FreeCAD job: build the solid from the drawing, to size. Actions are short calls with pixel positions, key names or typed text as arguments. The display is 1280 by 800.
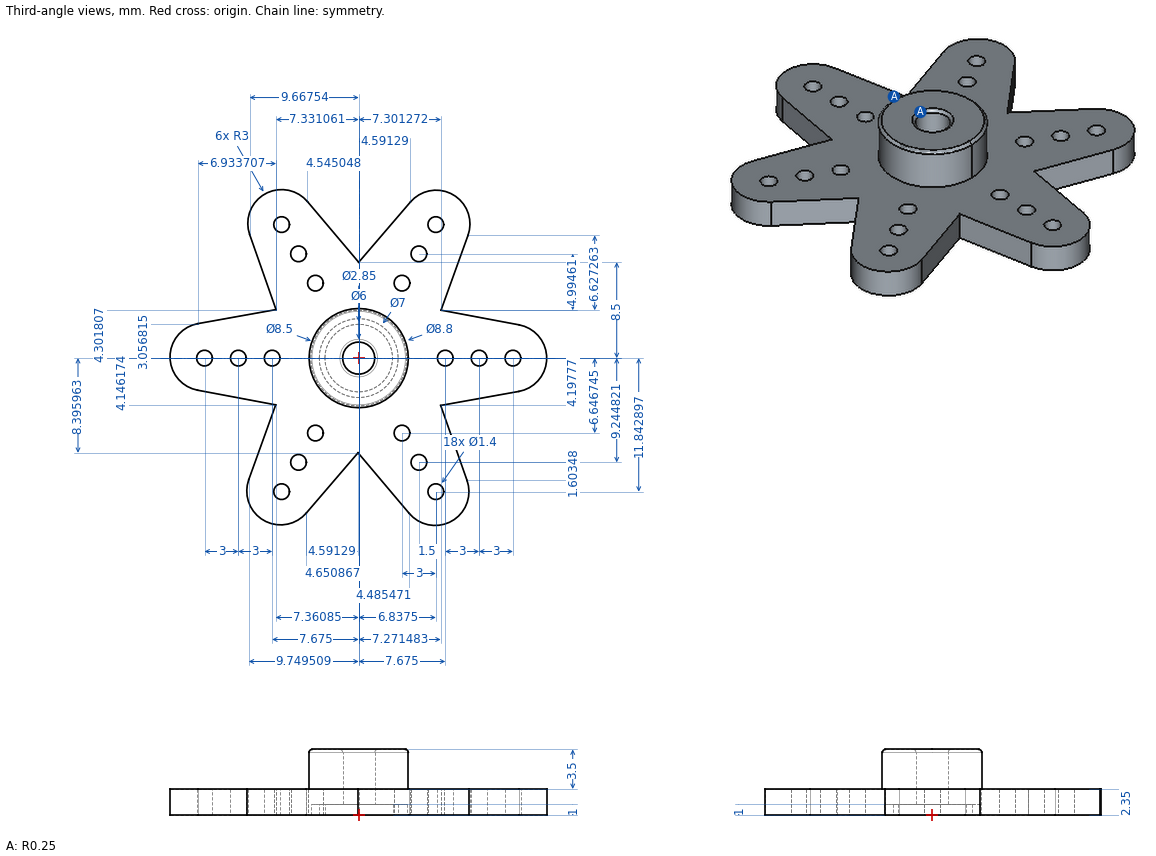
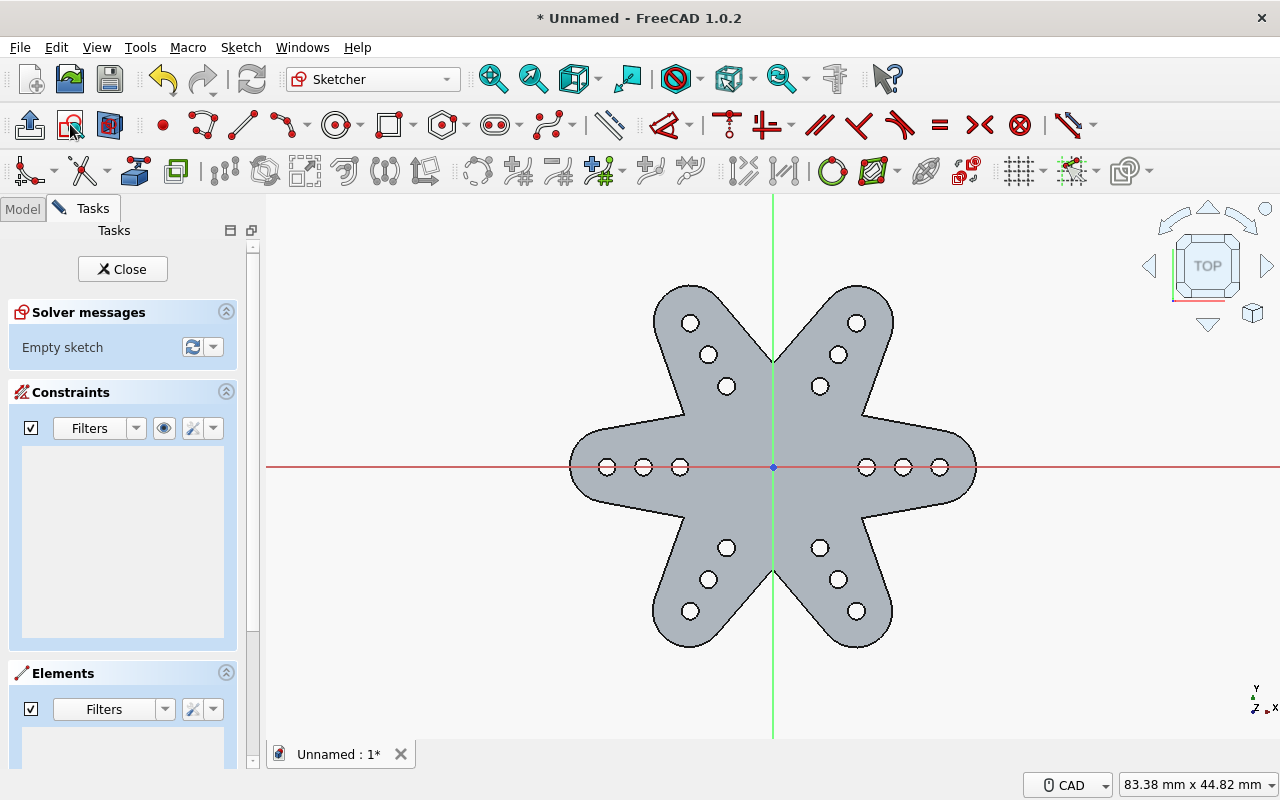
scroll(803, 467, up, 6)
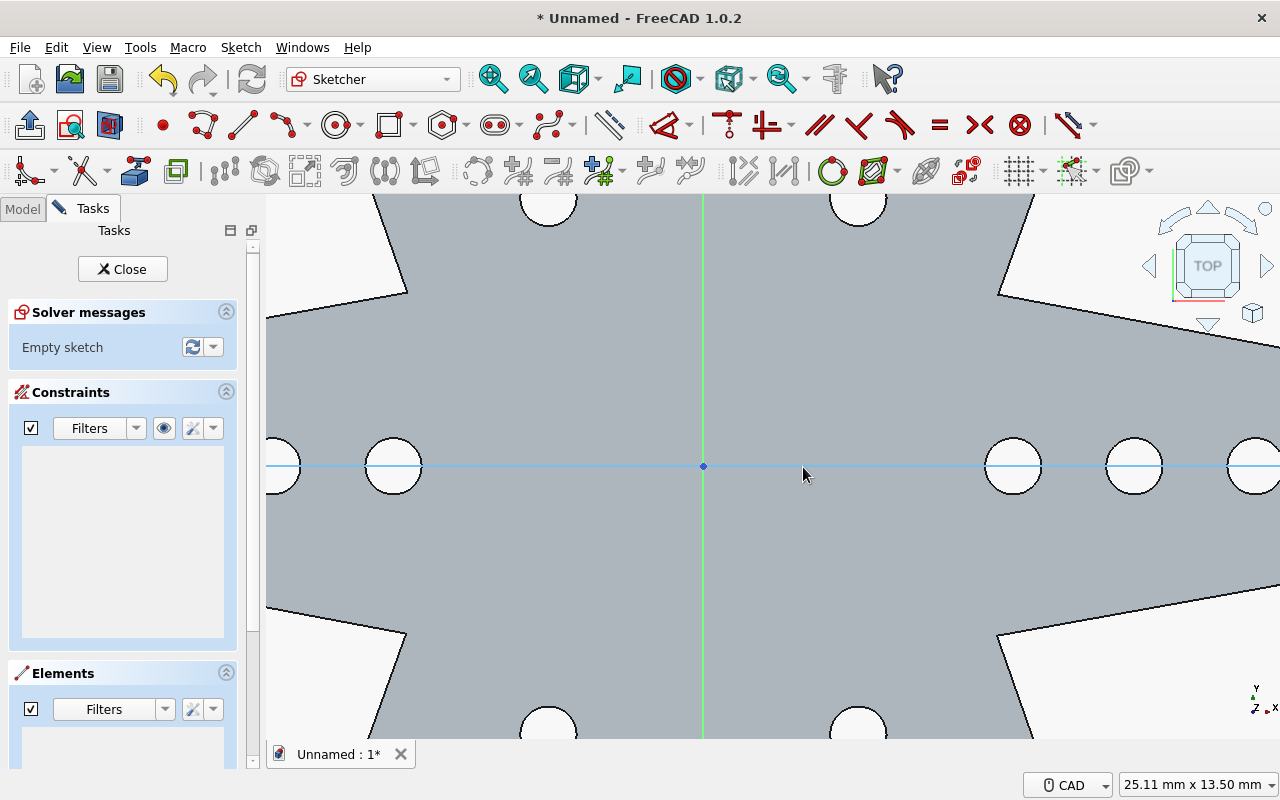
click(336, 126)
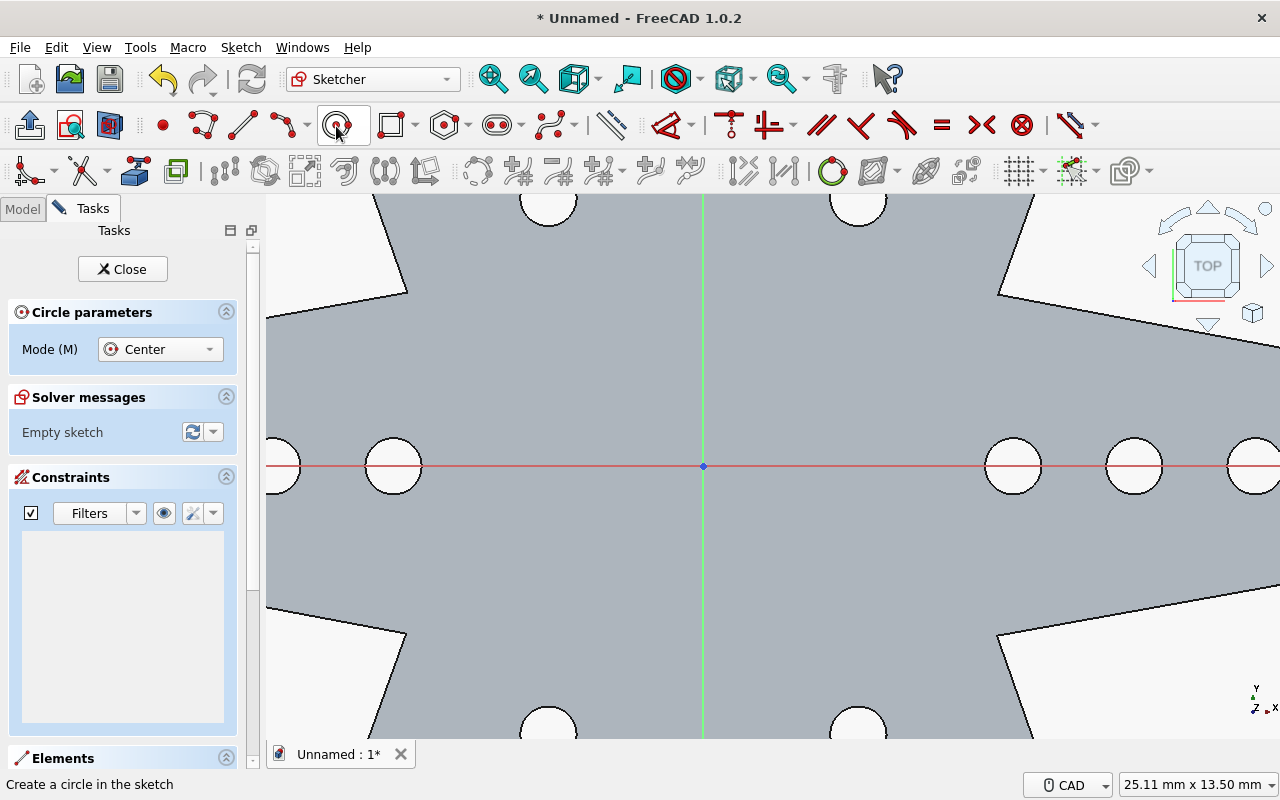
click(703, 466)
click(829, 341)
key(Escape)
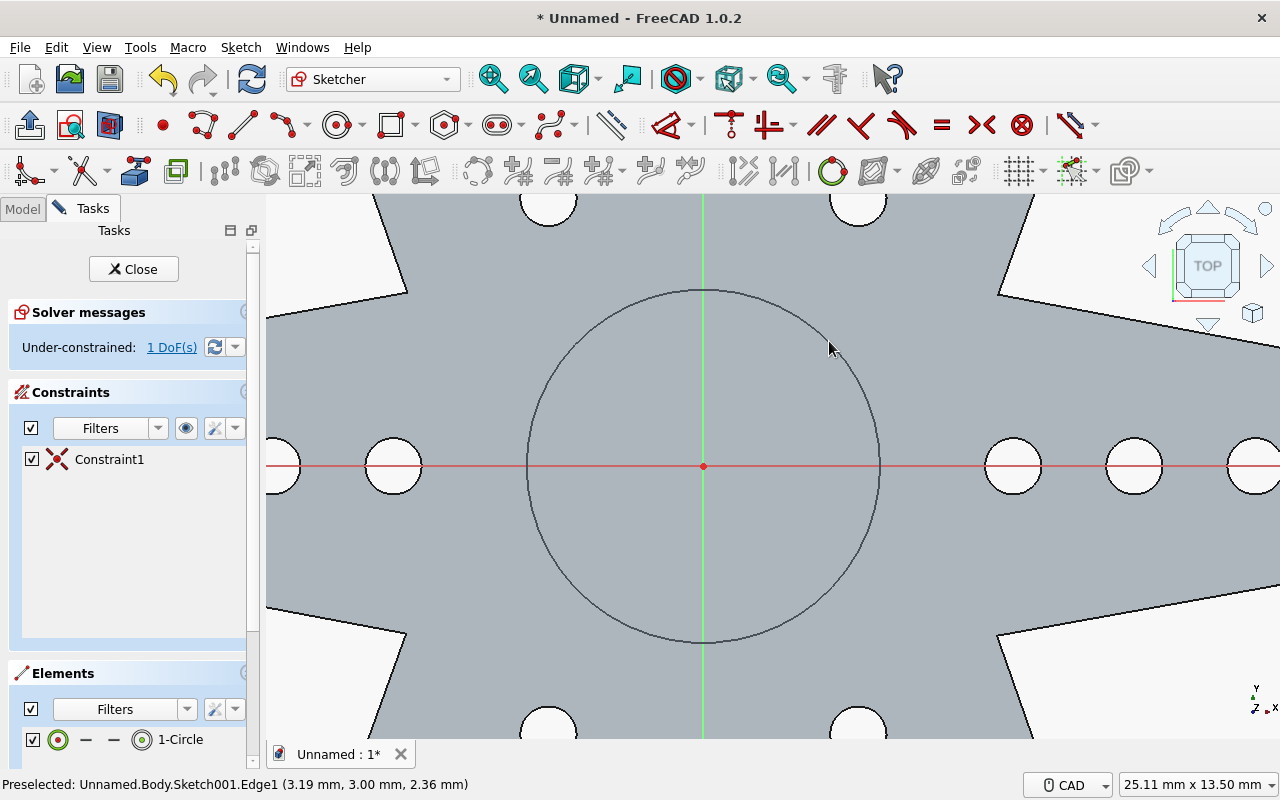
click(666, 126)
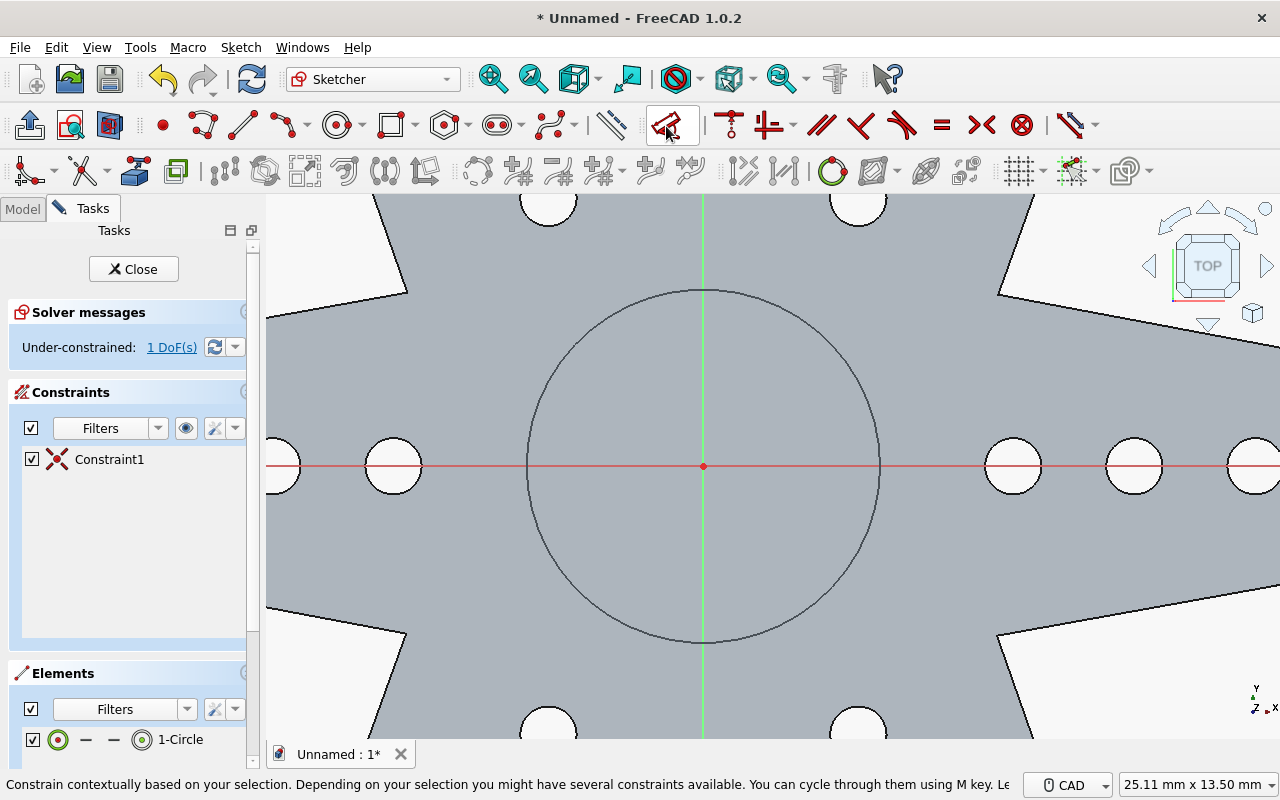
click(828, 341)
click(851, 318)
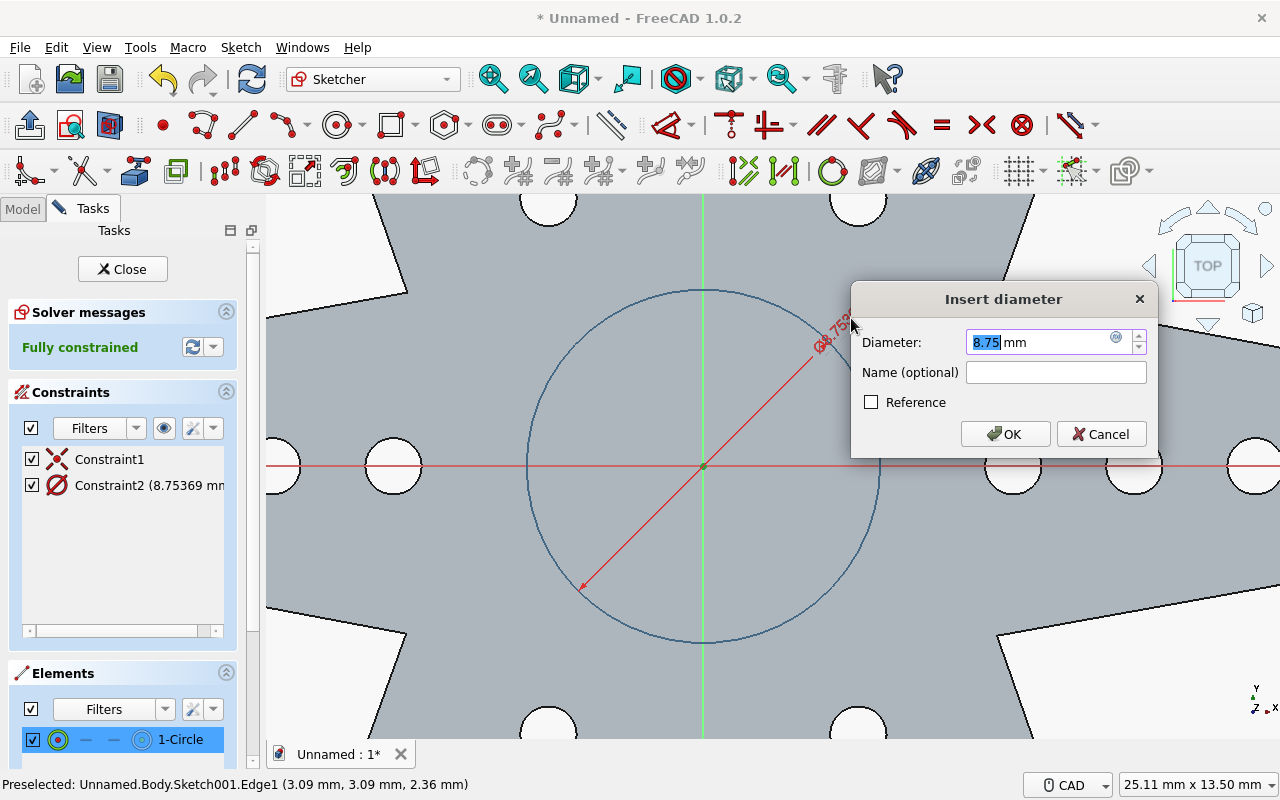
text(8.8)
key(Return)
key(Escape)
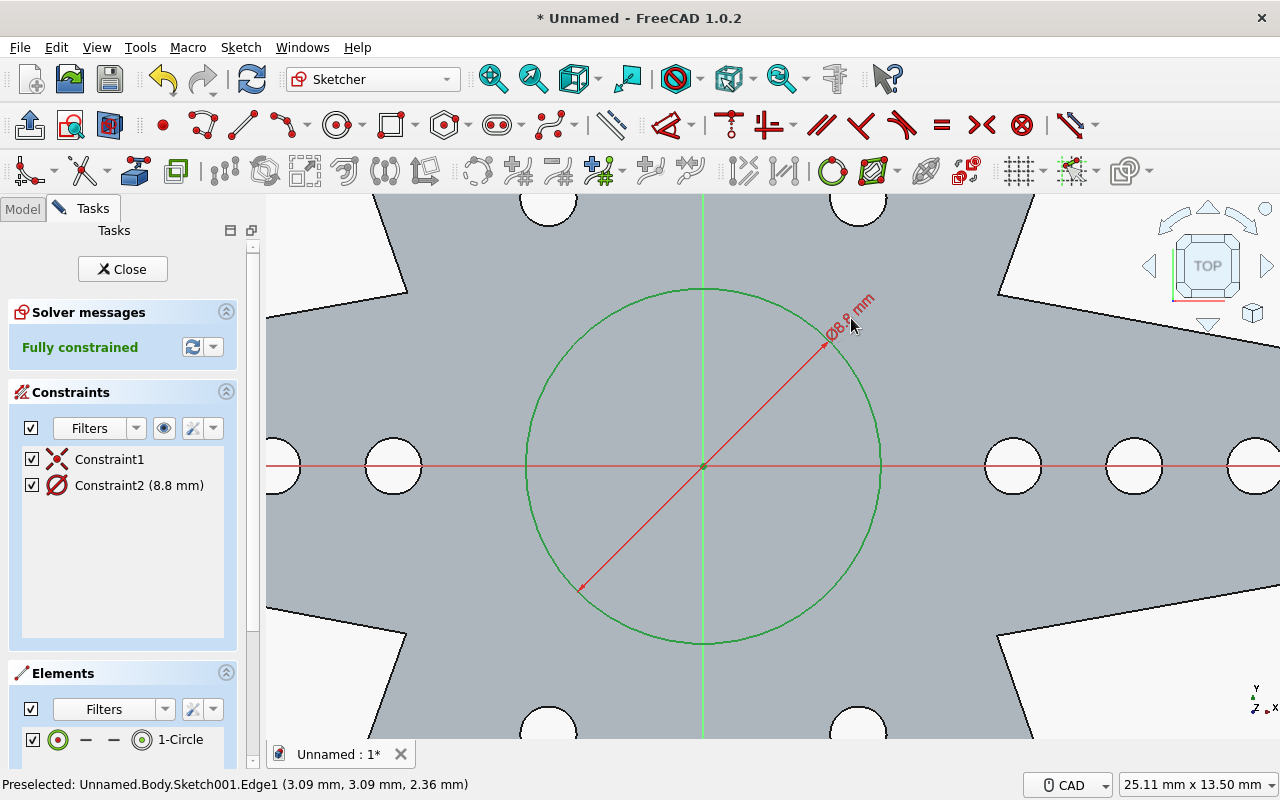
click(123, 269)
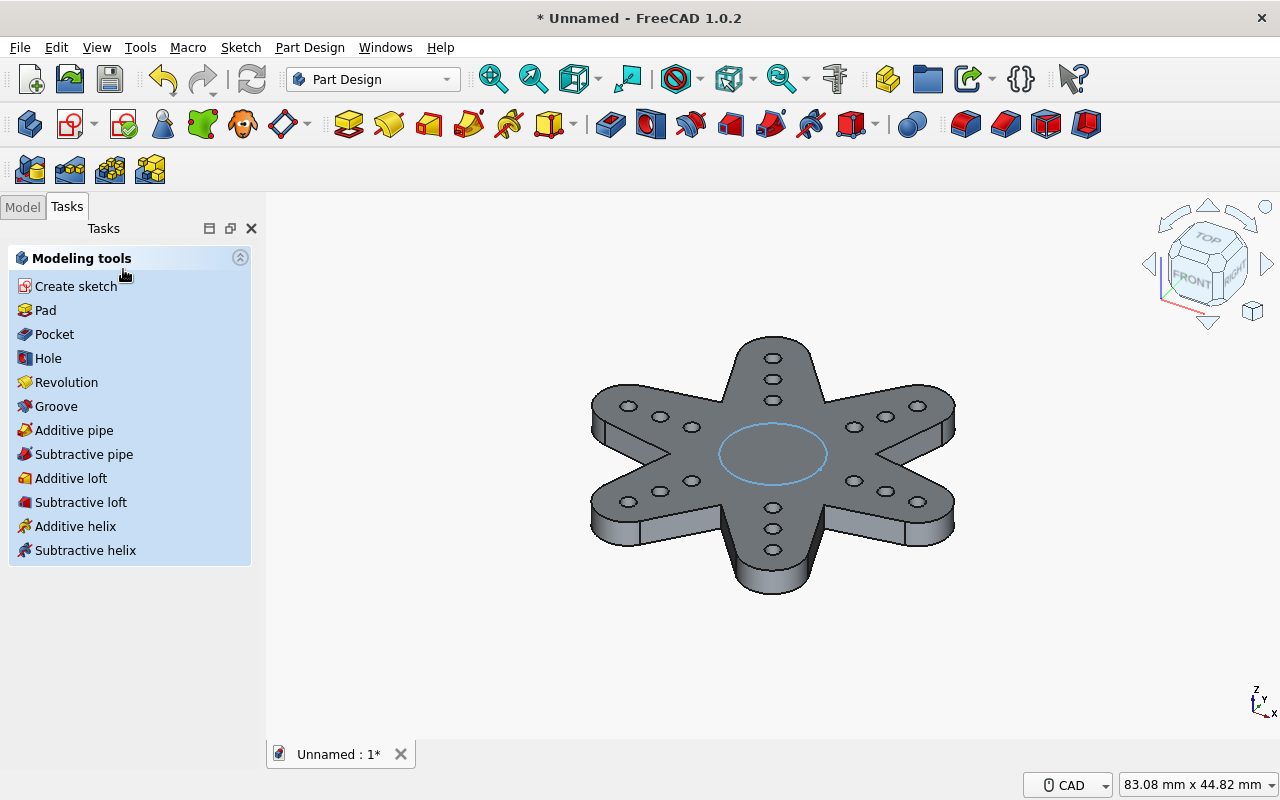
click(350, 124)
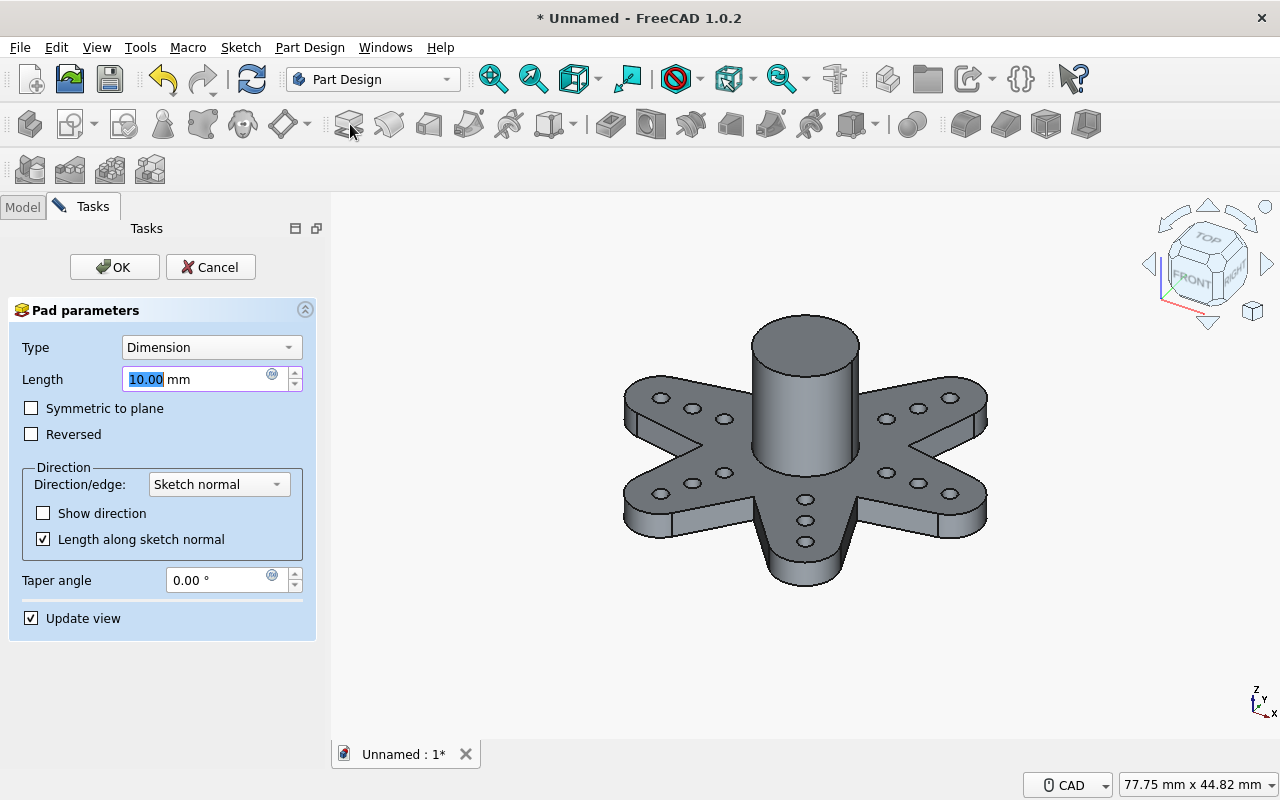
text(3.5)
key(Tab)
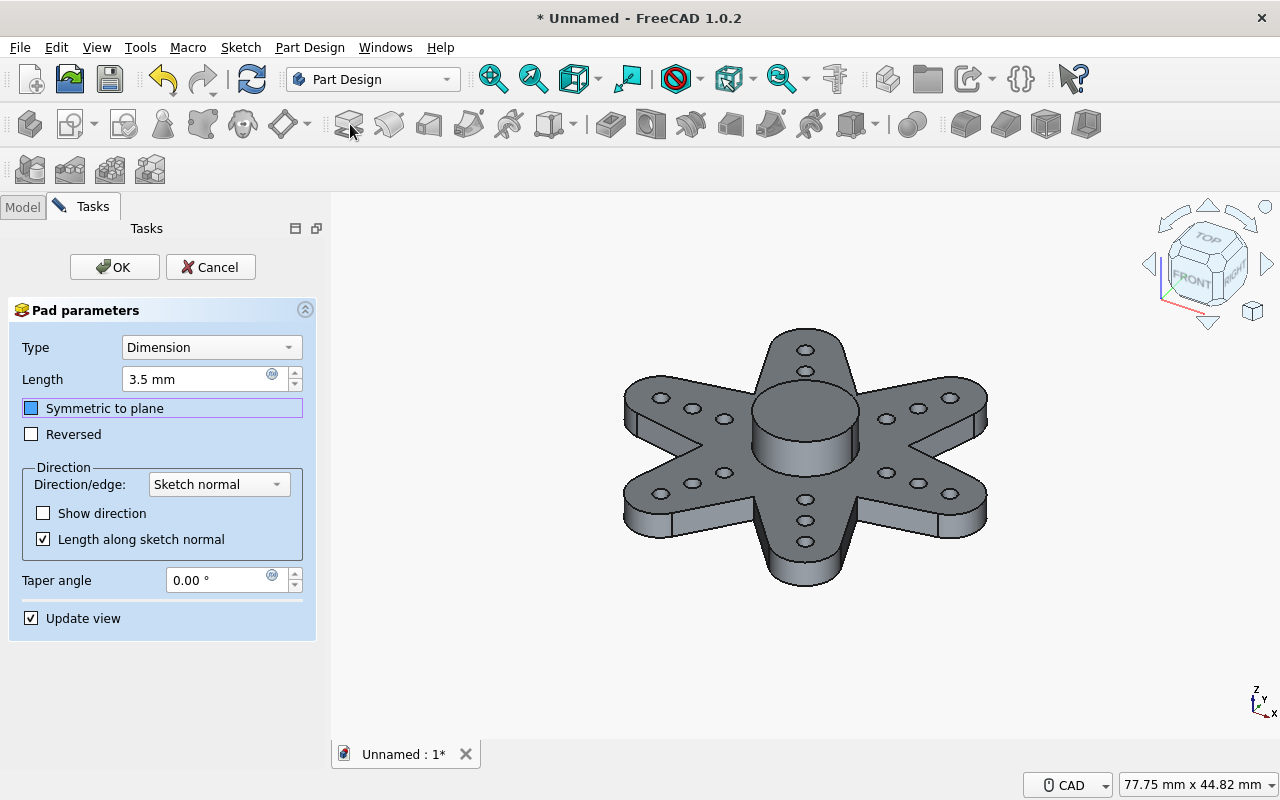
click(115, 267)